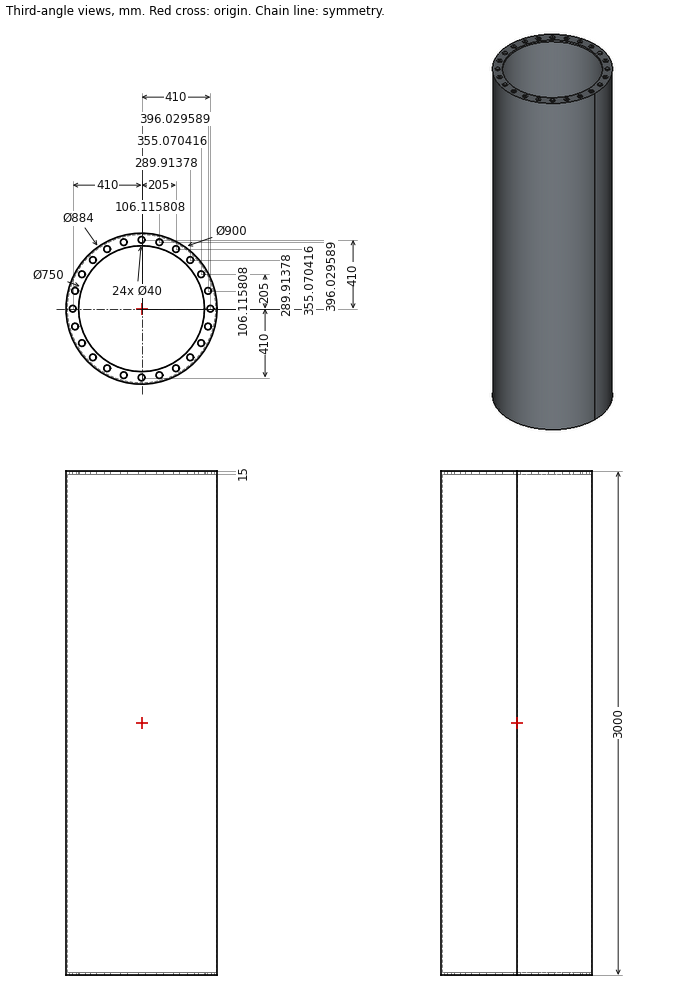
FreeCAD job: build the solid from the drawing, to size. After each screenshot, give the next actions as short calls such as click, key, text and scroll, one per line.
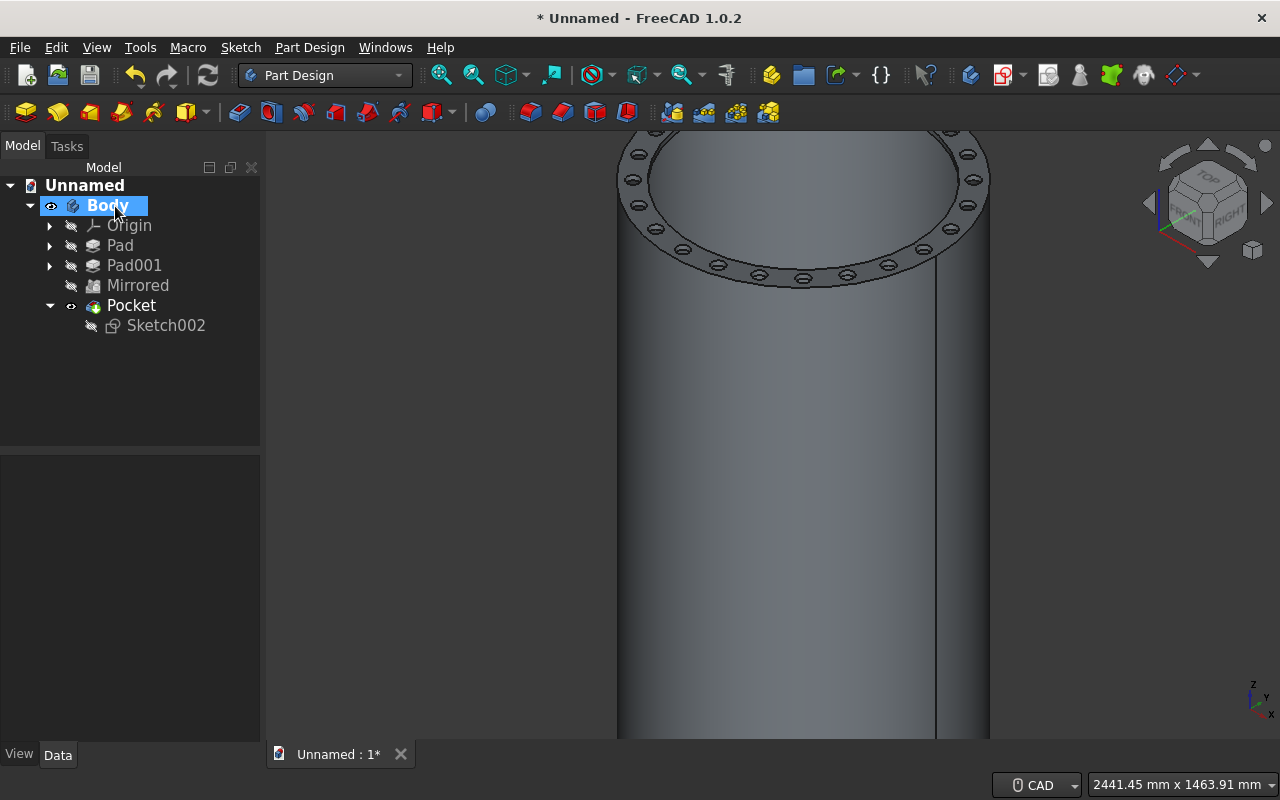
click(442, 76)